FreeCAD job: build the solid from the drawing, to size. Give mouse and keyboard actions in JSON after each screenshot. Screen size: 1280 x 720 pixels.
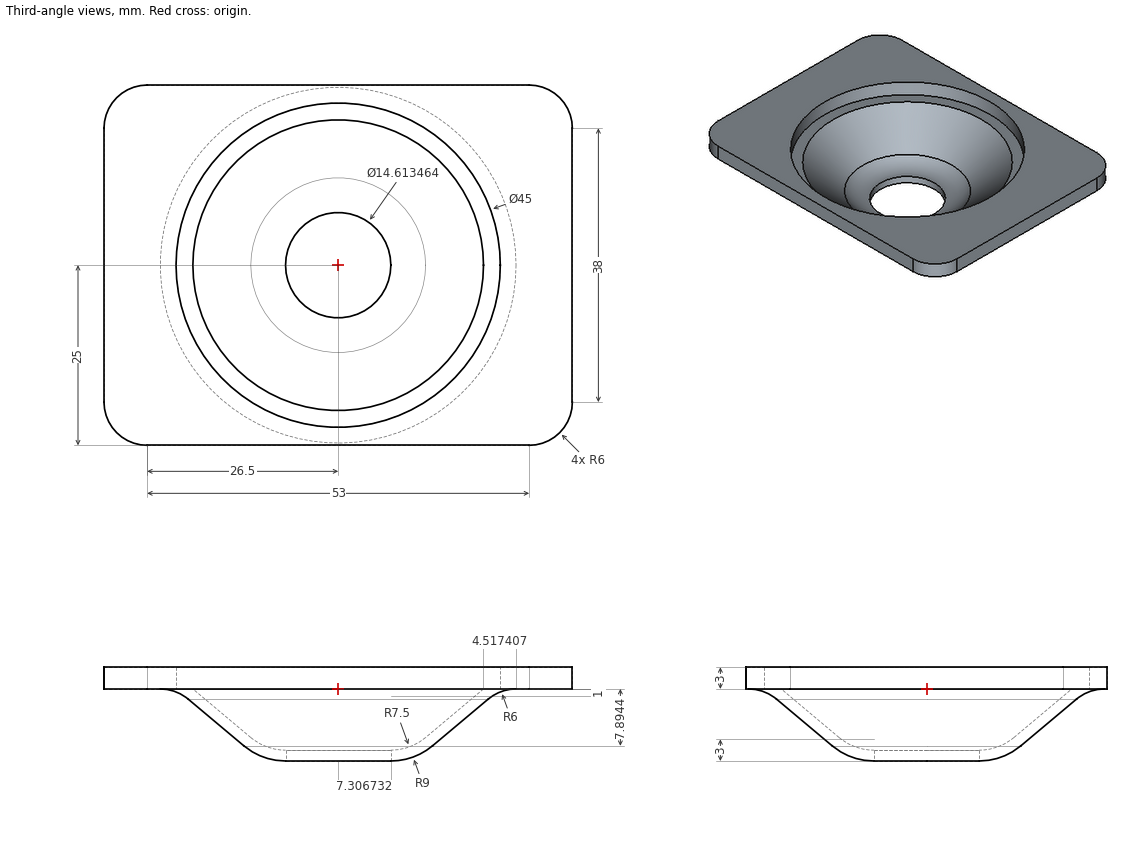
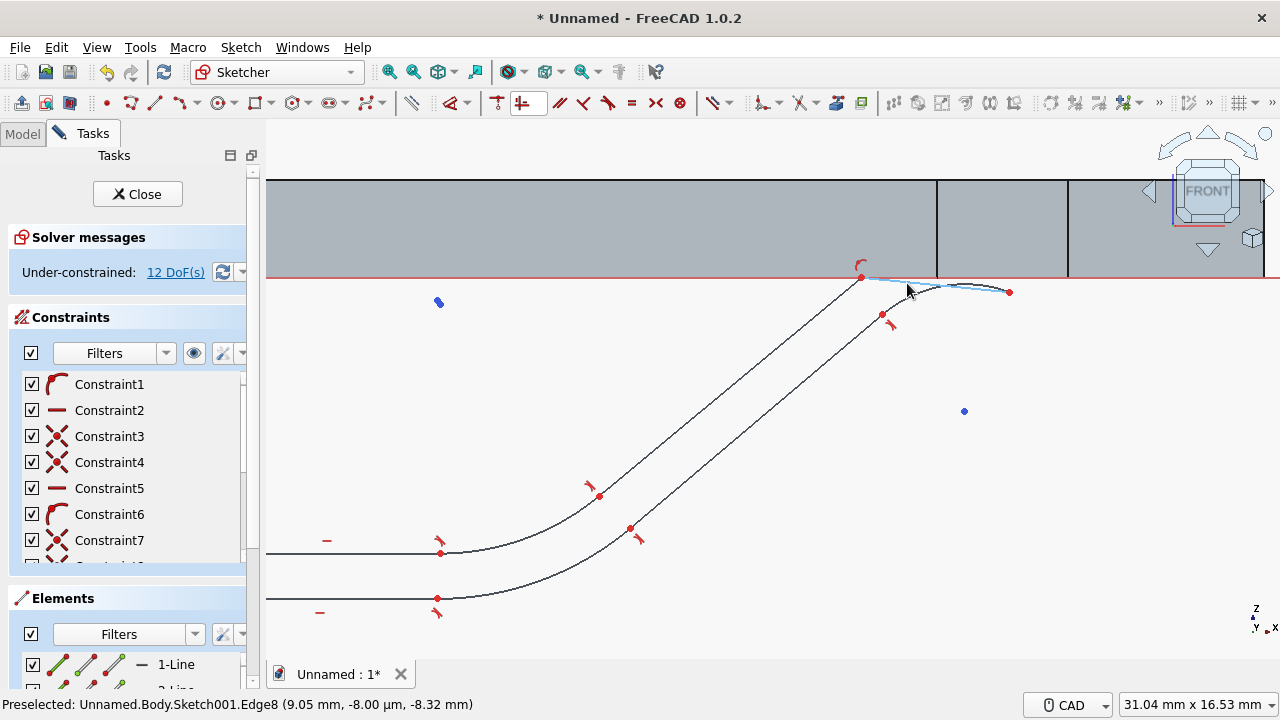
{"action": "left_click", "coordinate": [906, 282]}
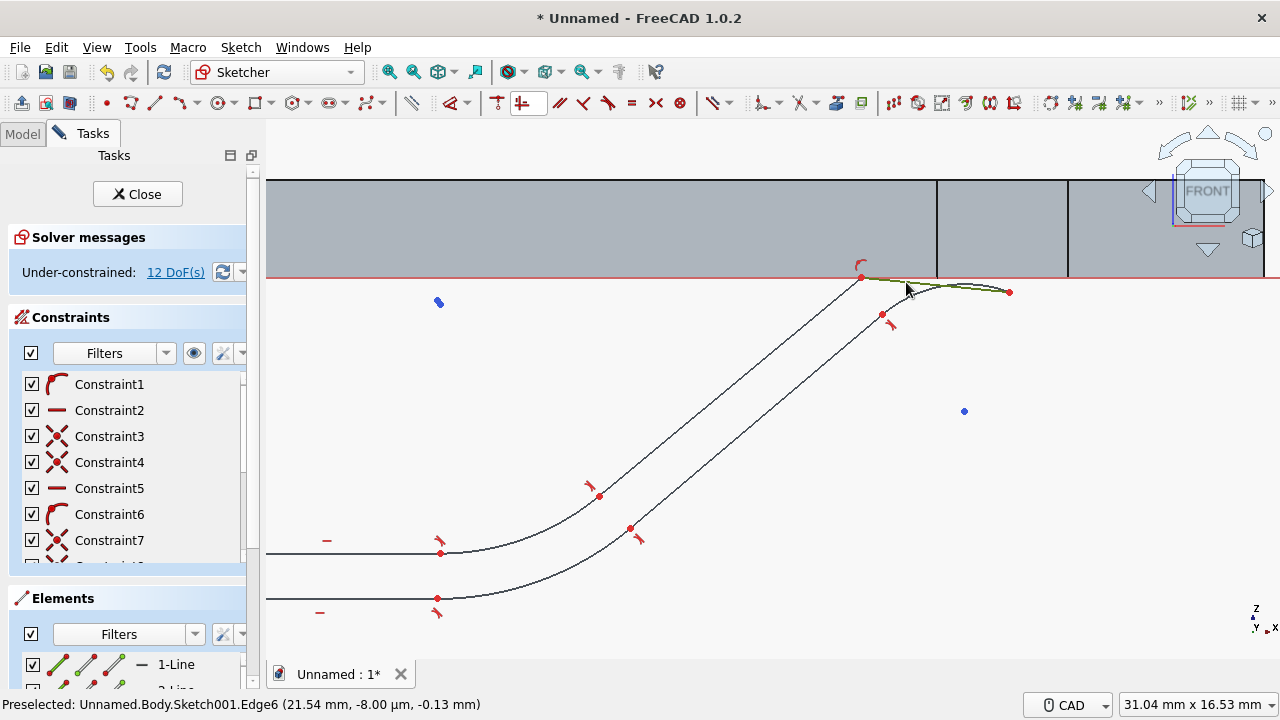
{"action": "scroll", "coordinate": [917, 294], "scroll_direction": "up", "scroll_amount": 2}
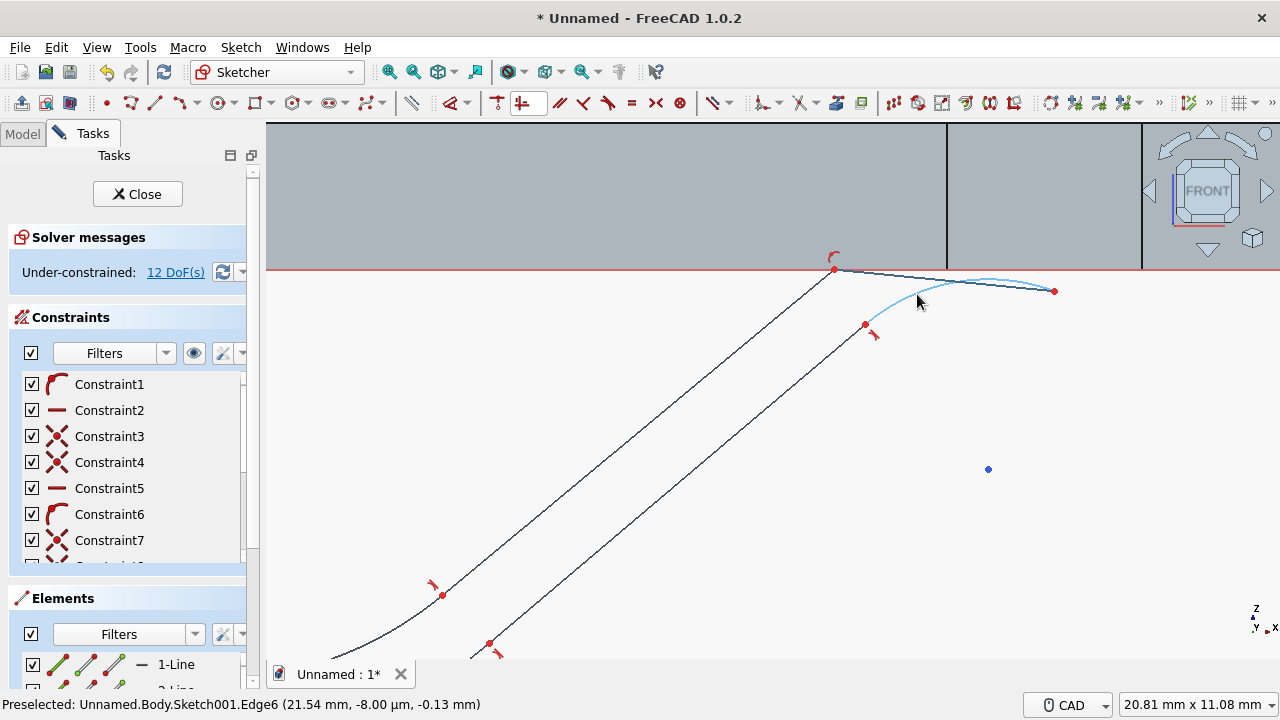
{"action": "left_click", "coordinate": [917, 293]}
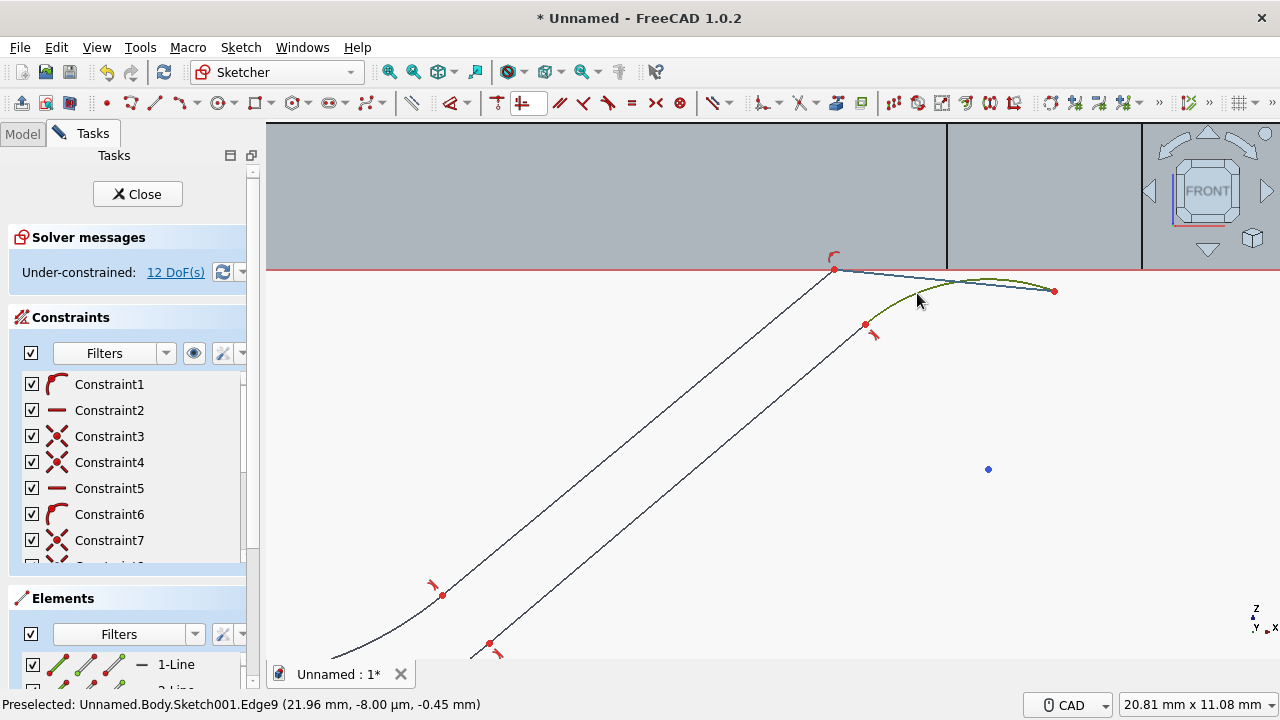
{"action": "key", "text": "t"}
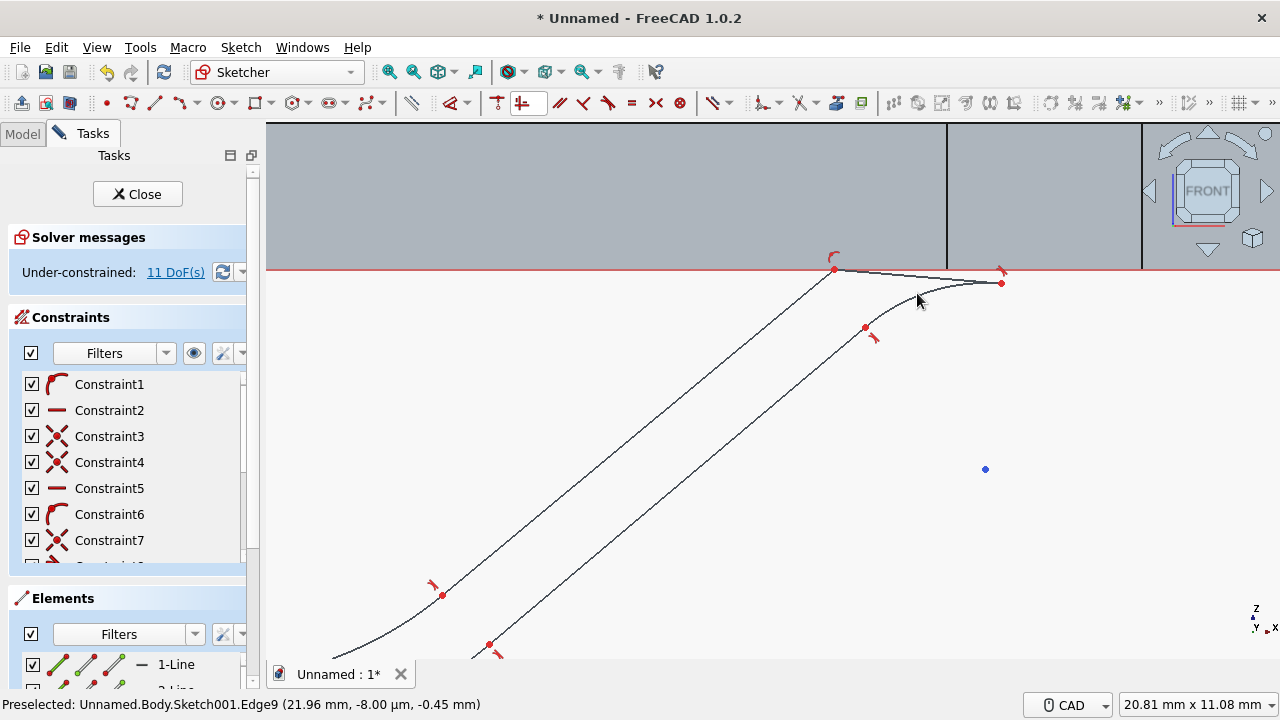
{"action": "scroll", "coordinate": [910, 288], "scroll_direction": "down", "scroll_amount": 4}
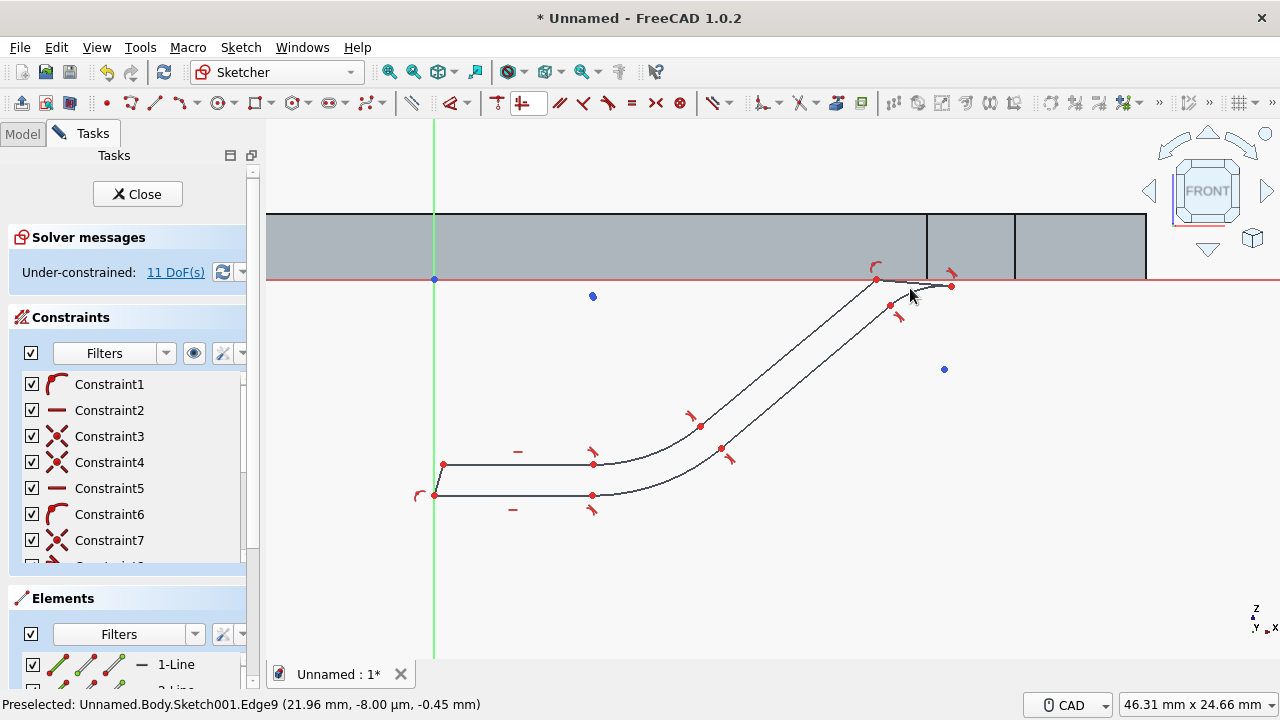
{"action": "scroll", "coordinate": [441, 474], "scroll_direction": "up", "scroll_amount": 4}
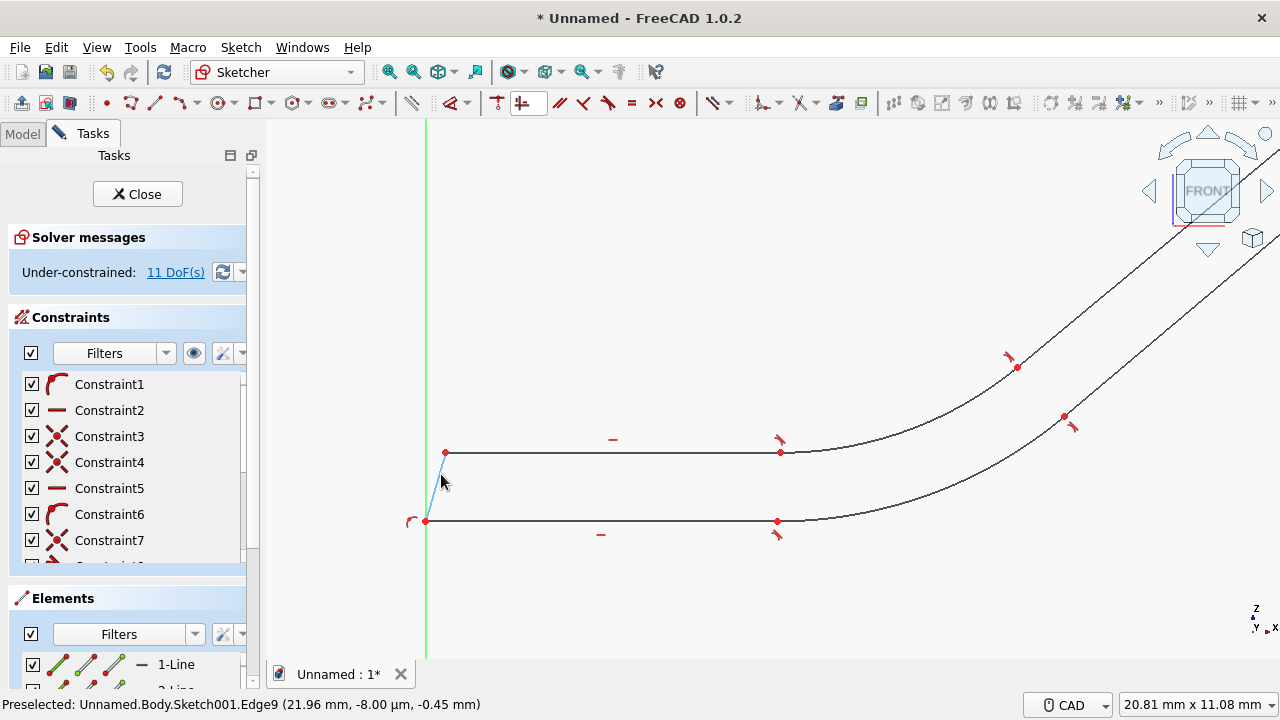
{"action": "left_click", "coordinate": [440, 473]}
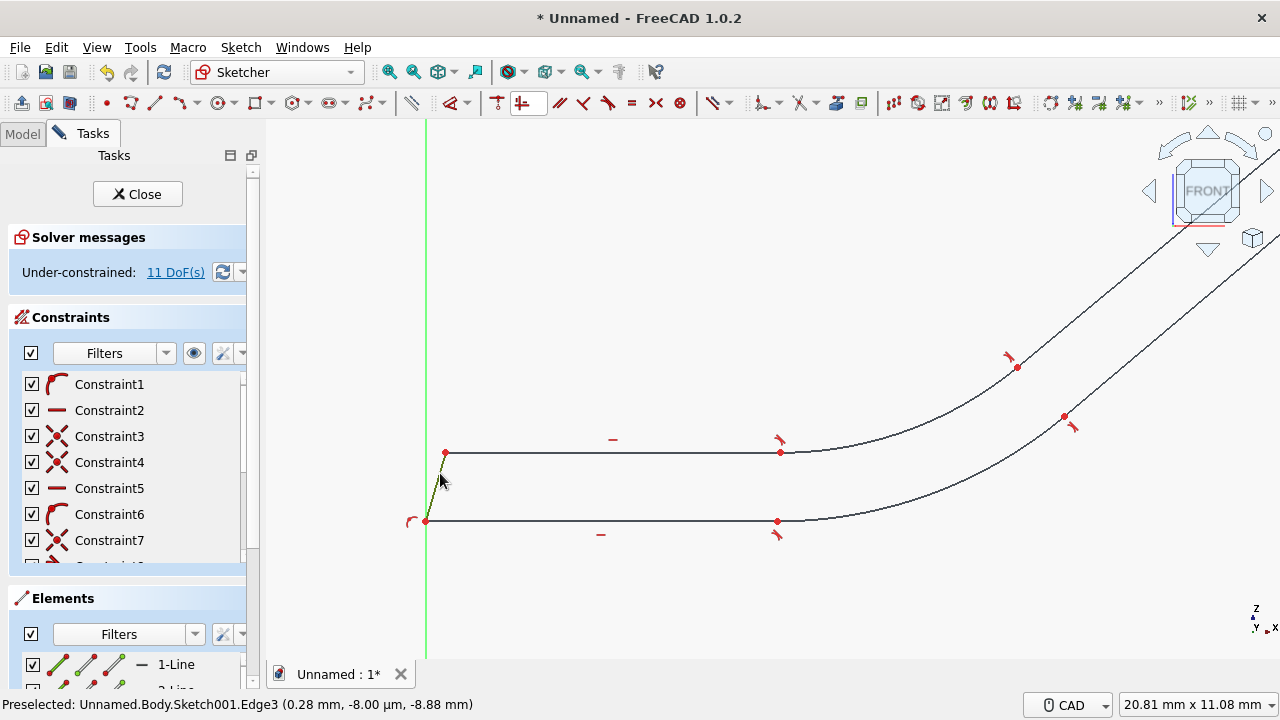
{"action": "key", "text": "v"}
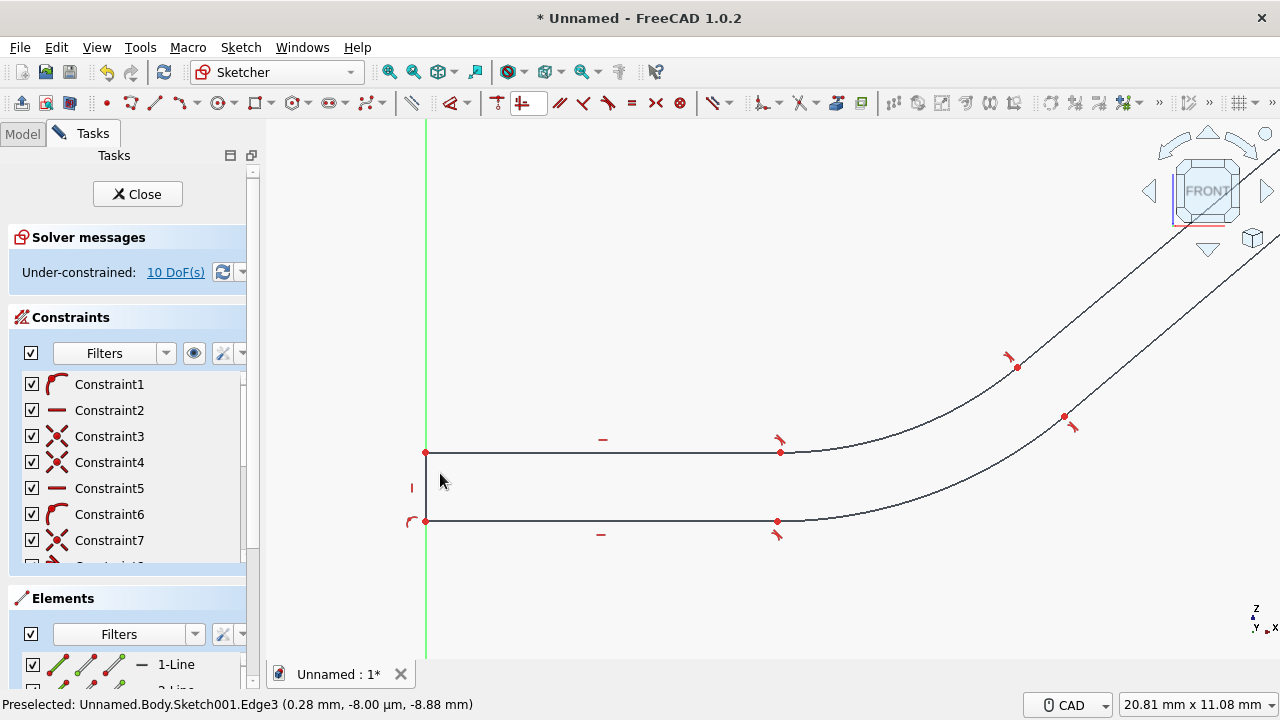
{"action": "scroll", "coordinate": [441, 474], "scroll_direction": "down", "scroll_amount": 4}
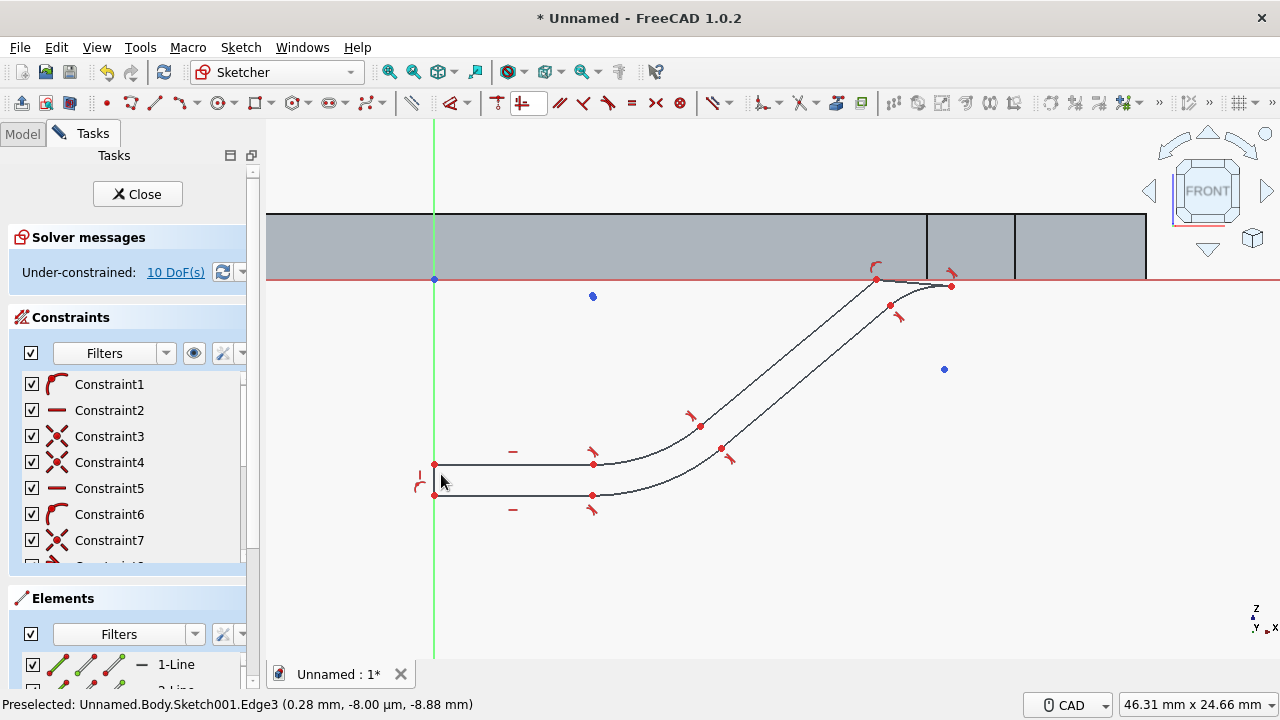
{"action": "left_click", "coordinate": [891, 281]}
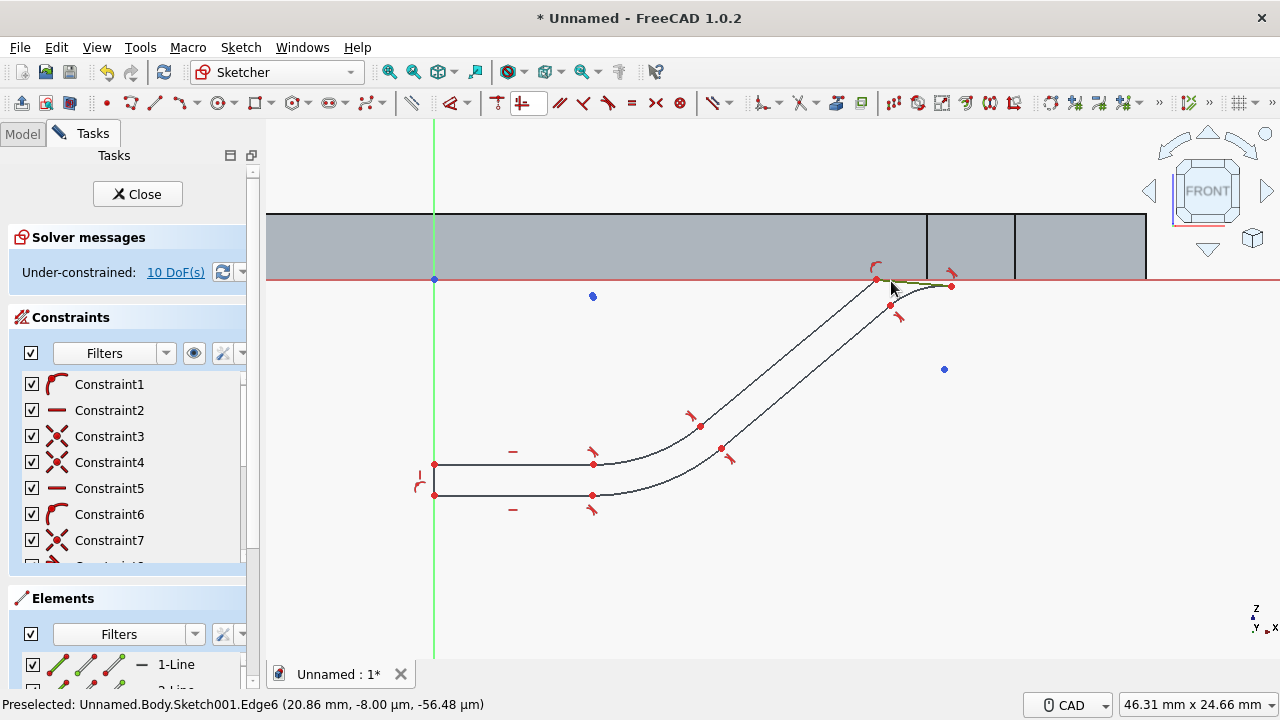
{"action": "key", "text": "h"}